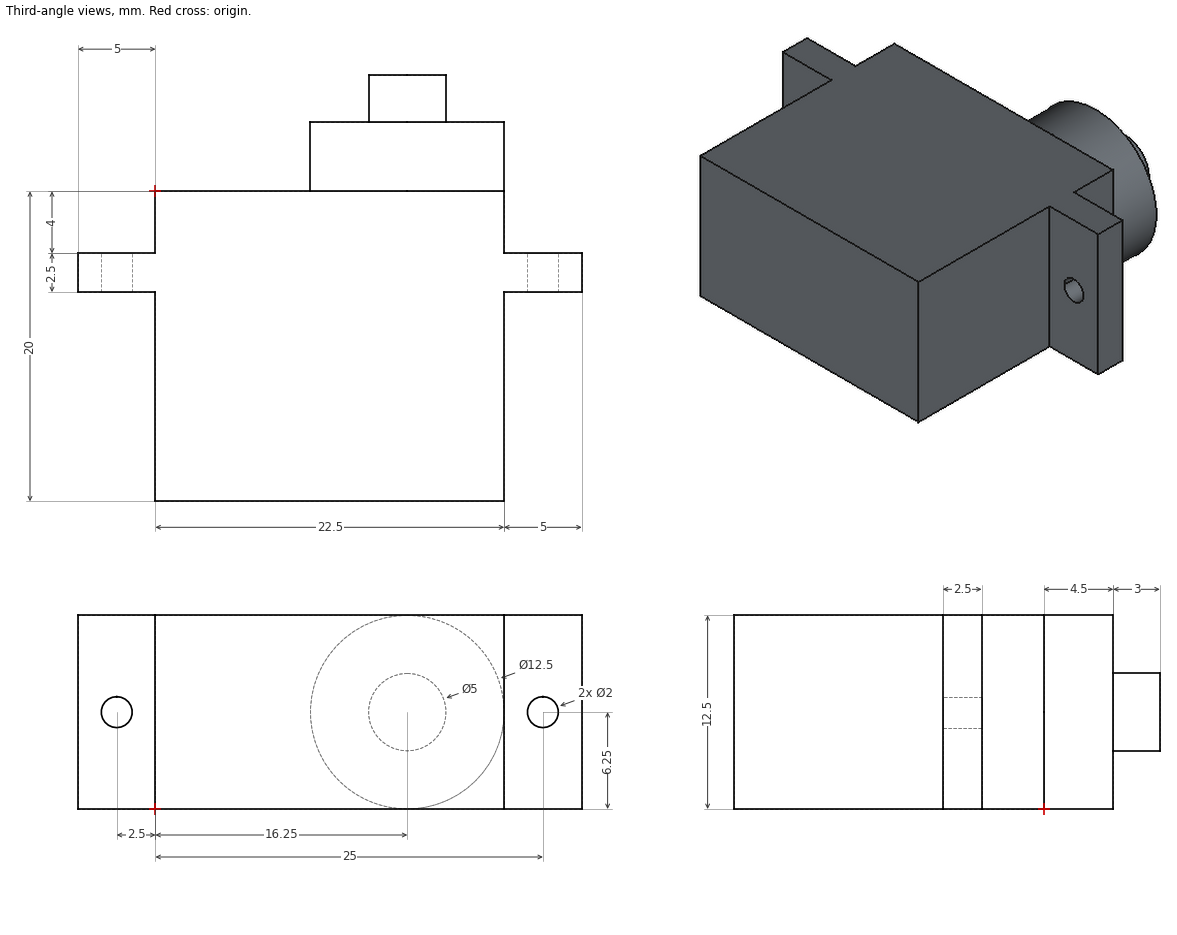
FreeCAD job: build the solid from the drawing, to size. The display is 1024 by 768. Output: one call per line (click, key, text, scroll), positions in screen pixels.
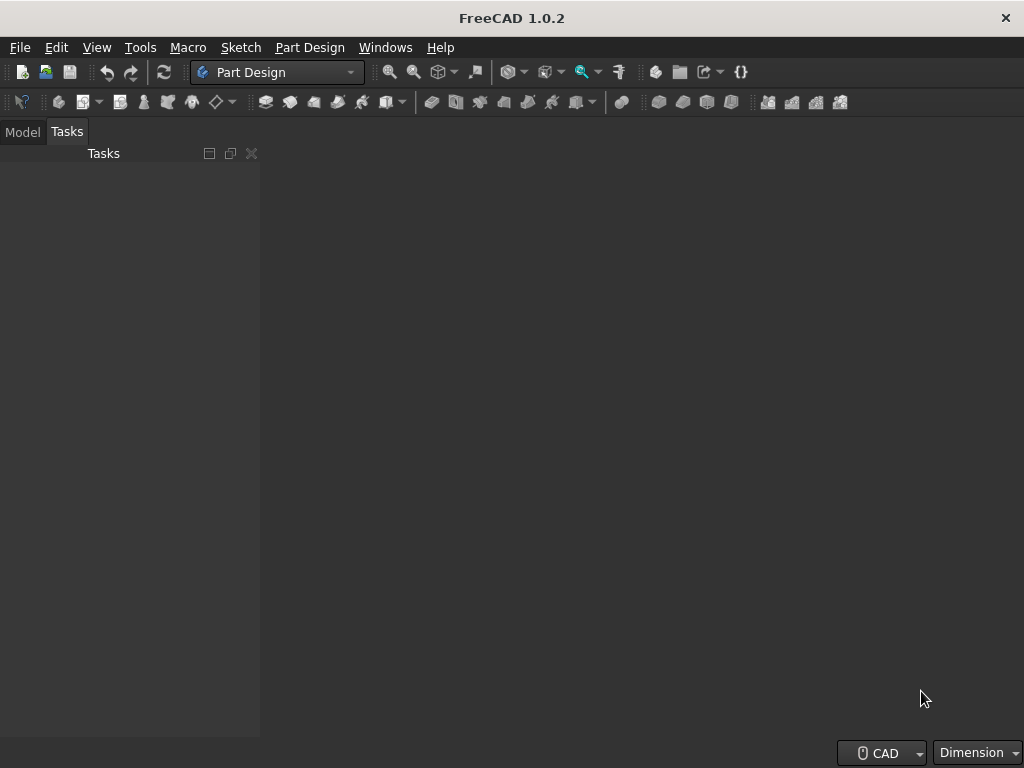
key(ctrl+n)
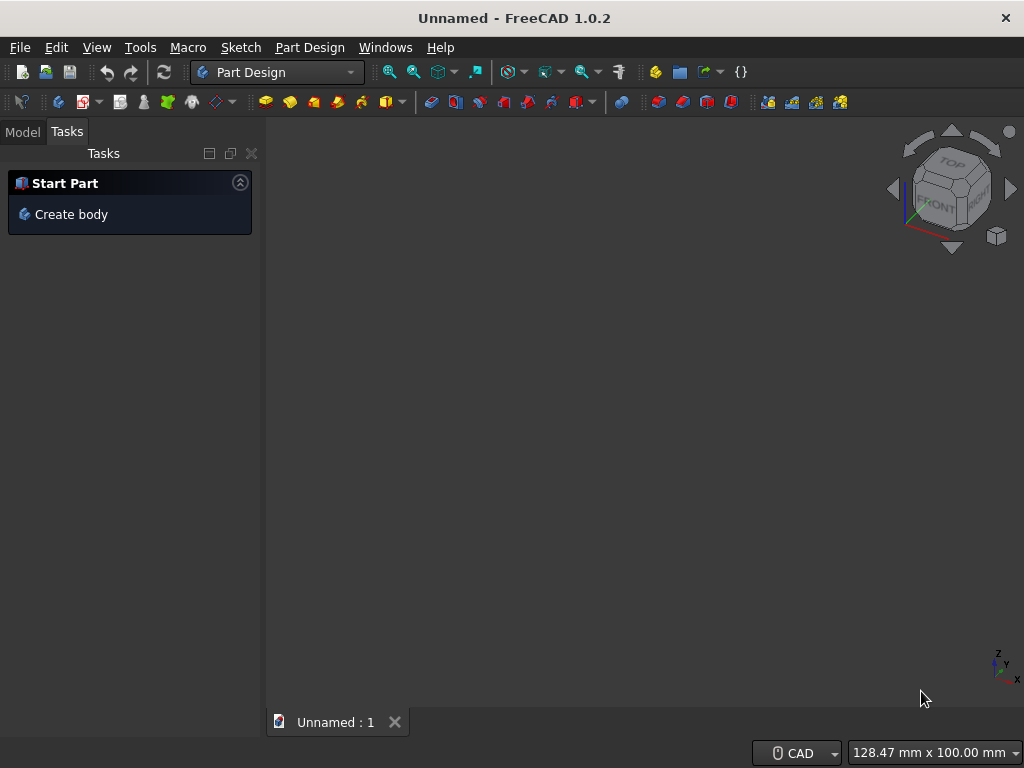
click(84, 102)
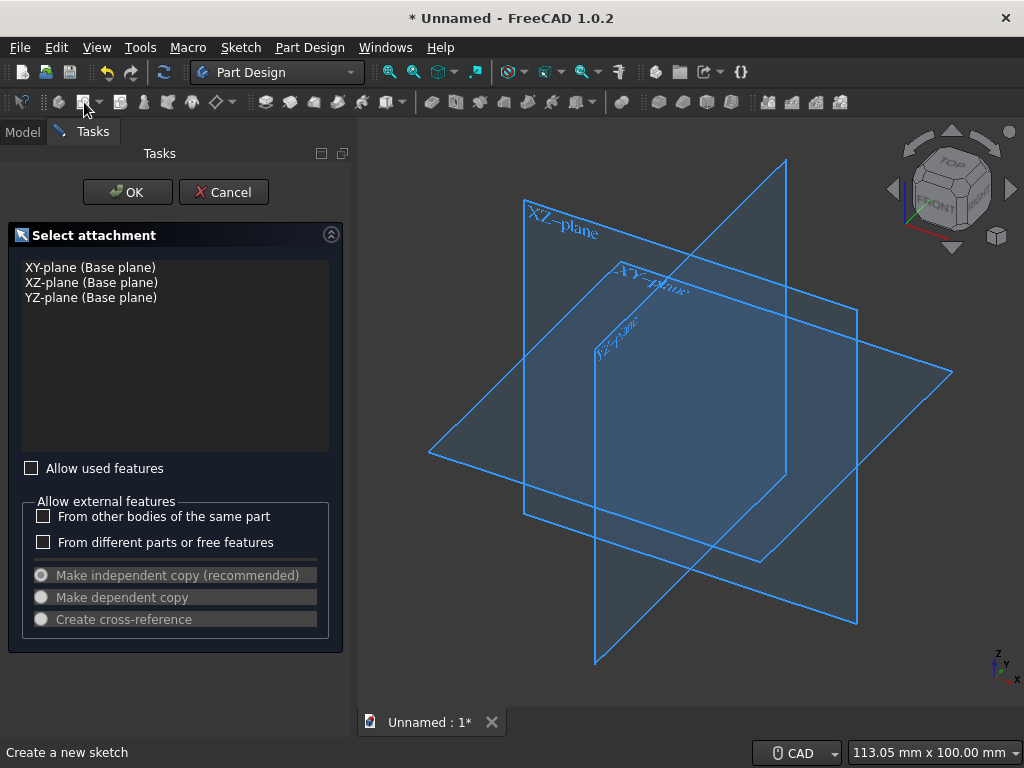
click(82, 268)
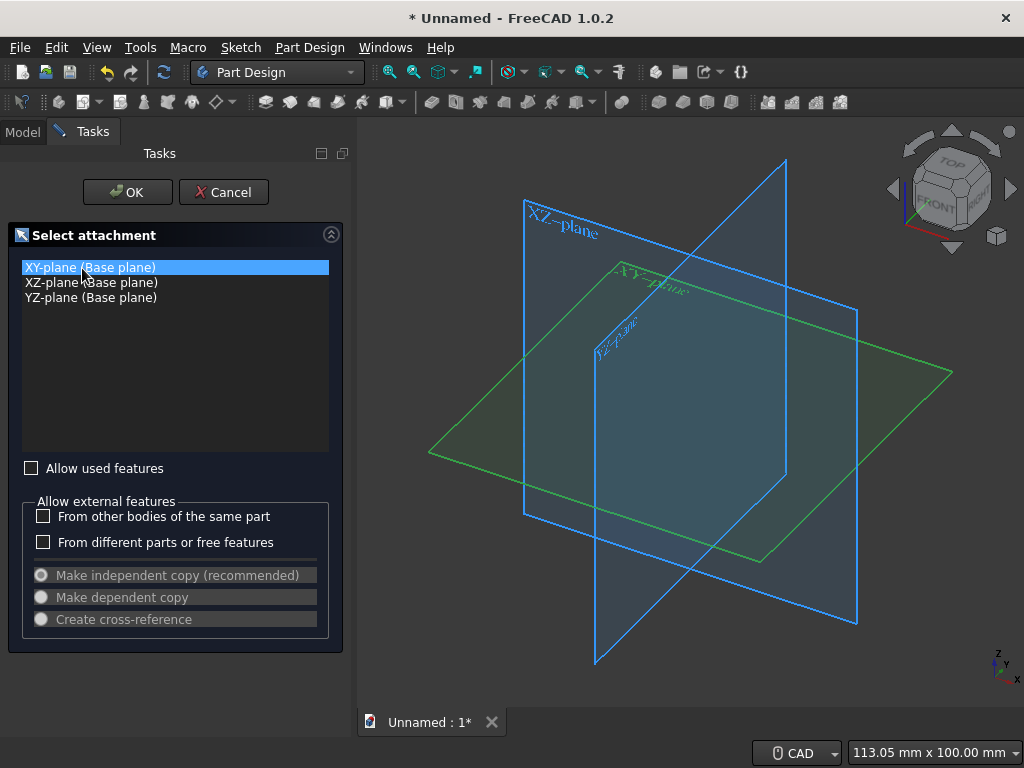
click(128, 192)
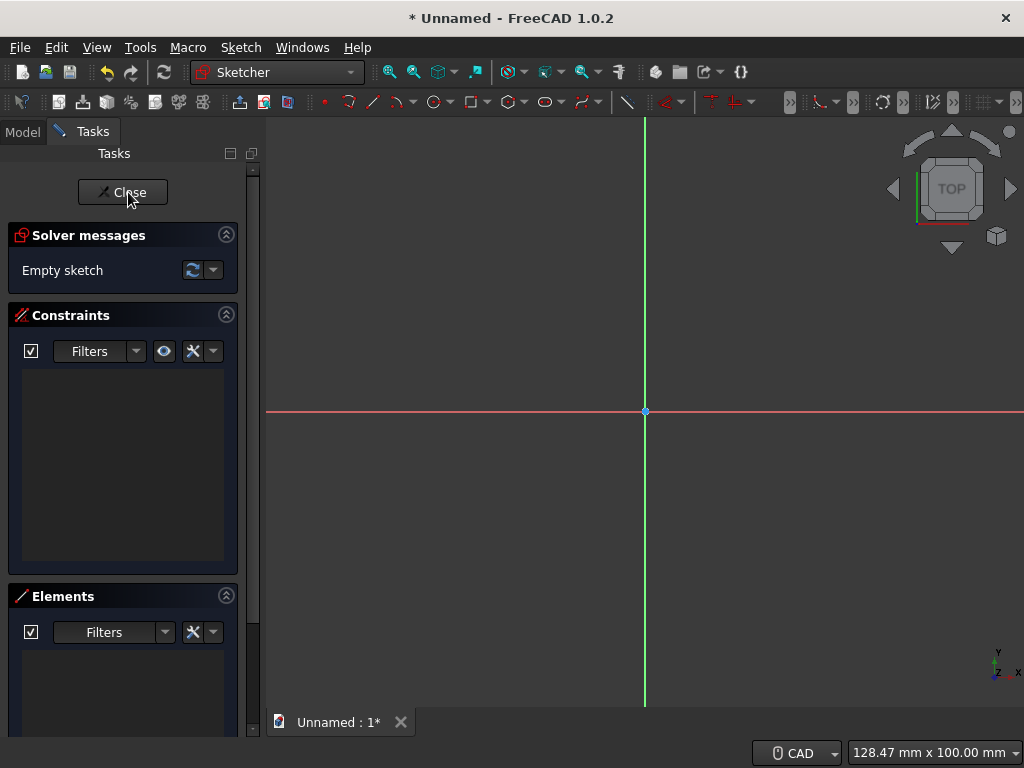
scroll(821, 519, up, 4)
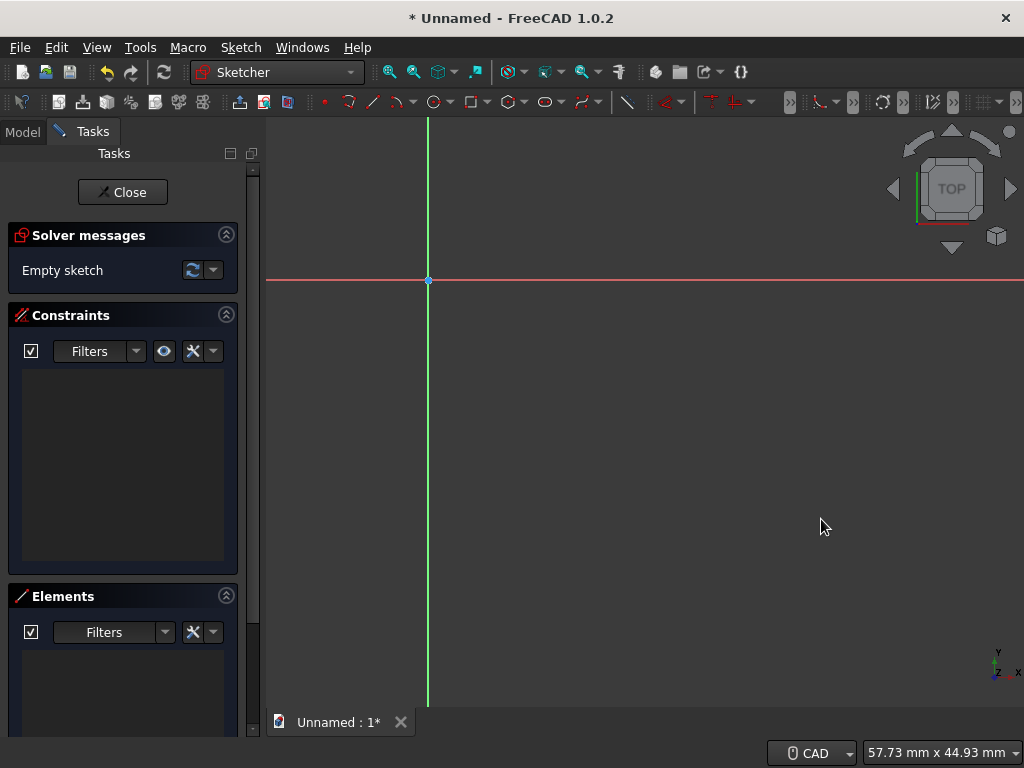
key(g)
key(m)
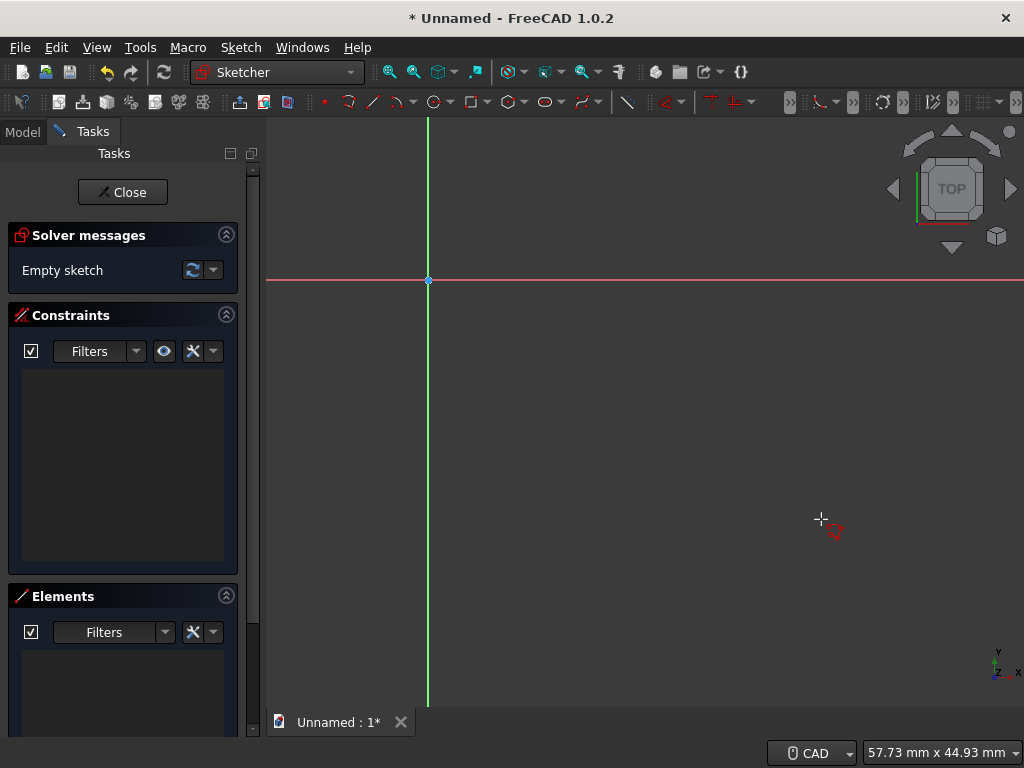
click(428, 280)
click(437, 333)
click(363, 333)
click(363, 365)
click(428, 365)
click(437, 543)
click(724, 543)
click(724, 365)
click(790, 365)
click(790, 333)
click(724, 333)
click(724, 289)
click(428, 280)
key(Escape)
key(Escape)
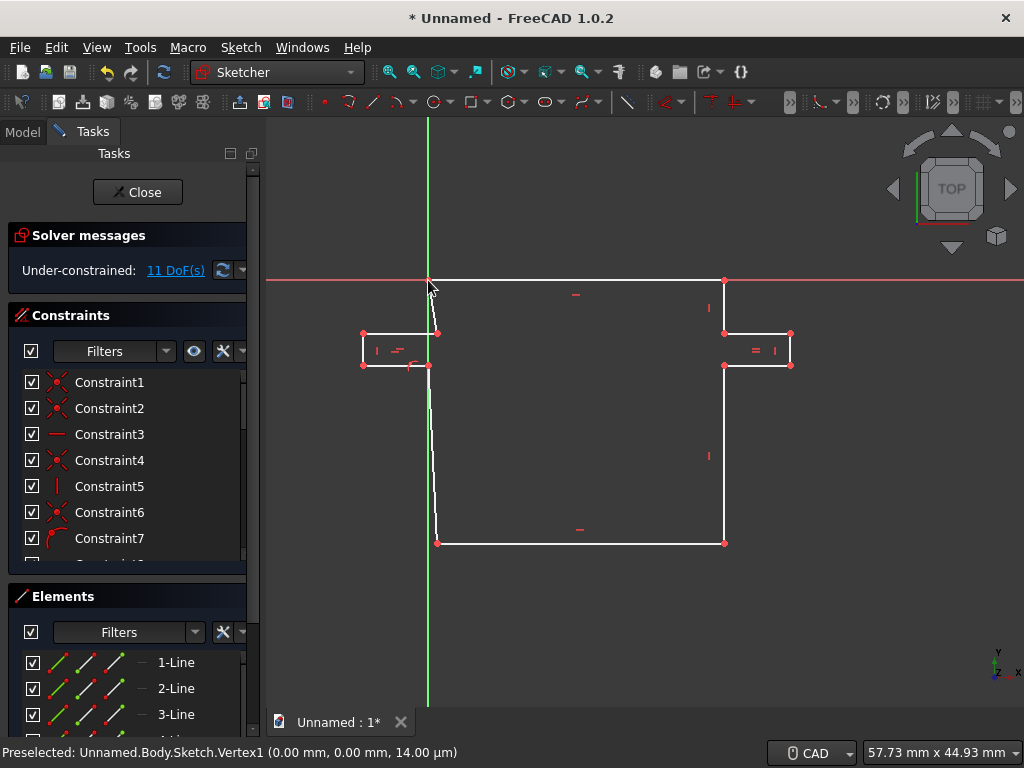
click(431, 296)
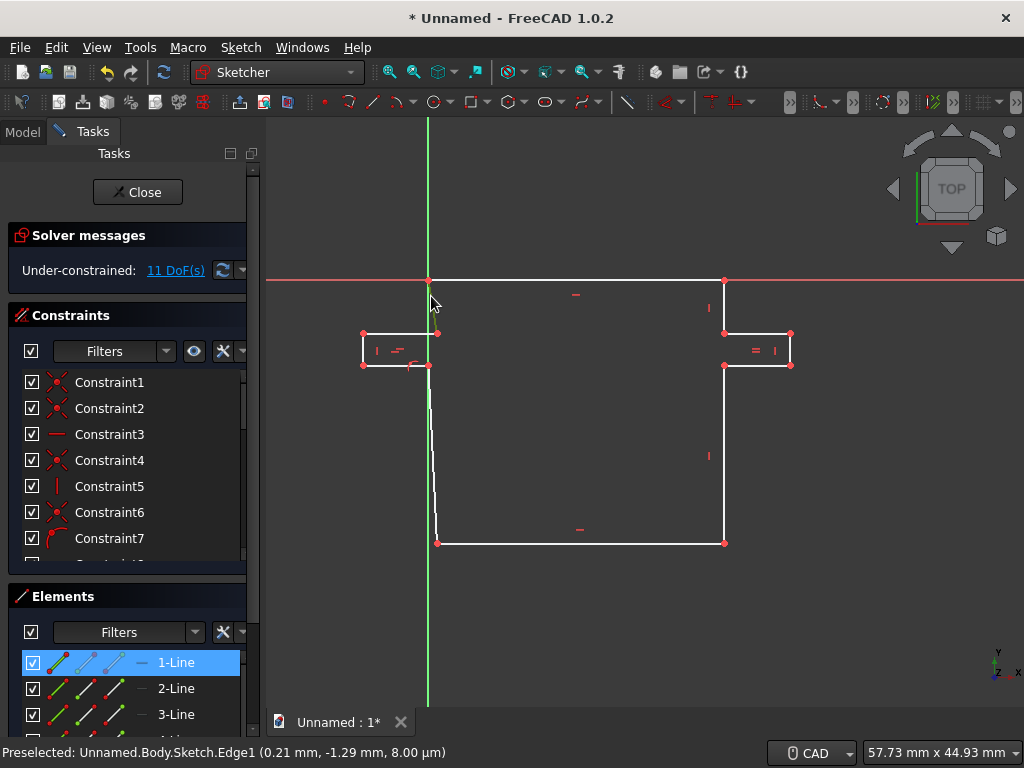
key(v)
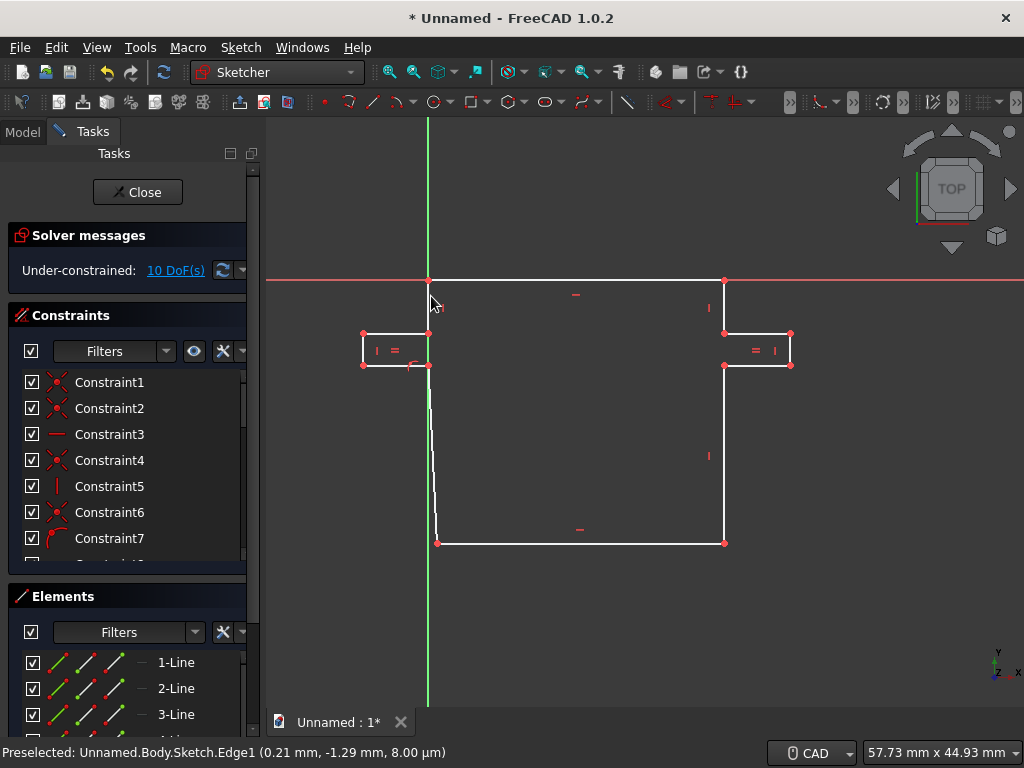
click(431, 419)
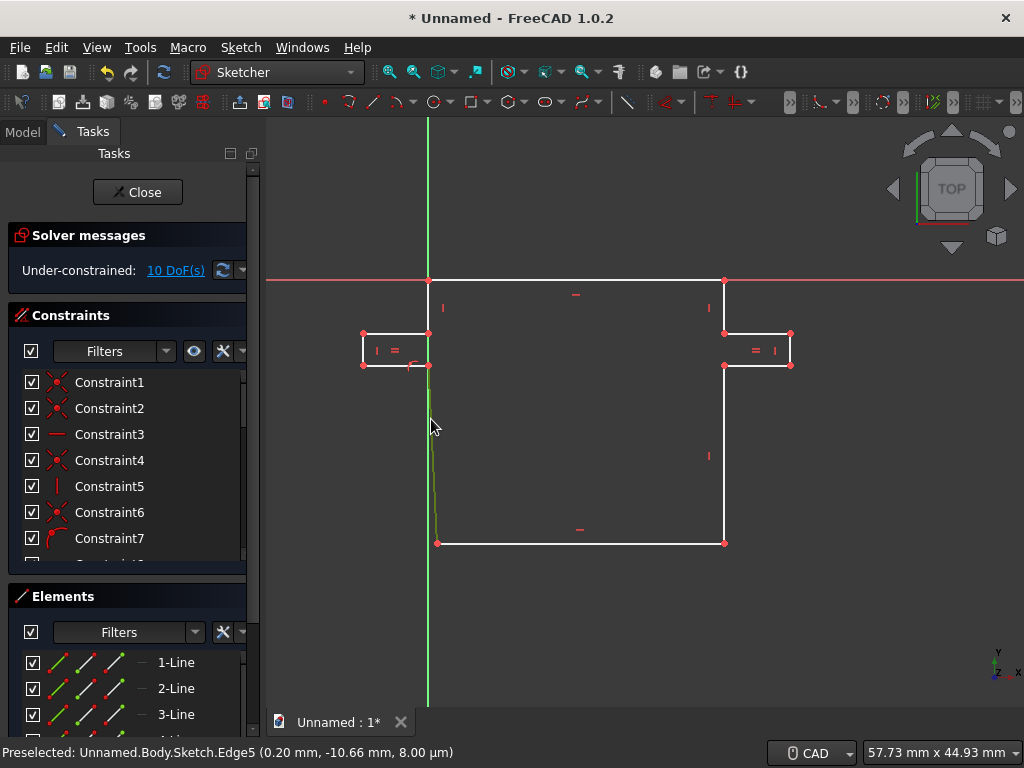
key(v)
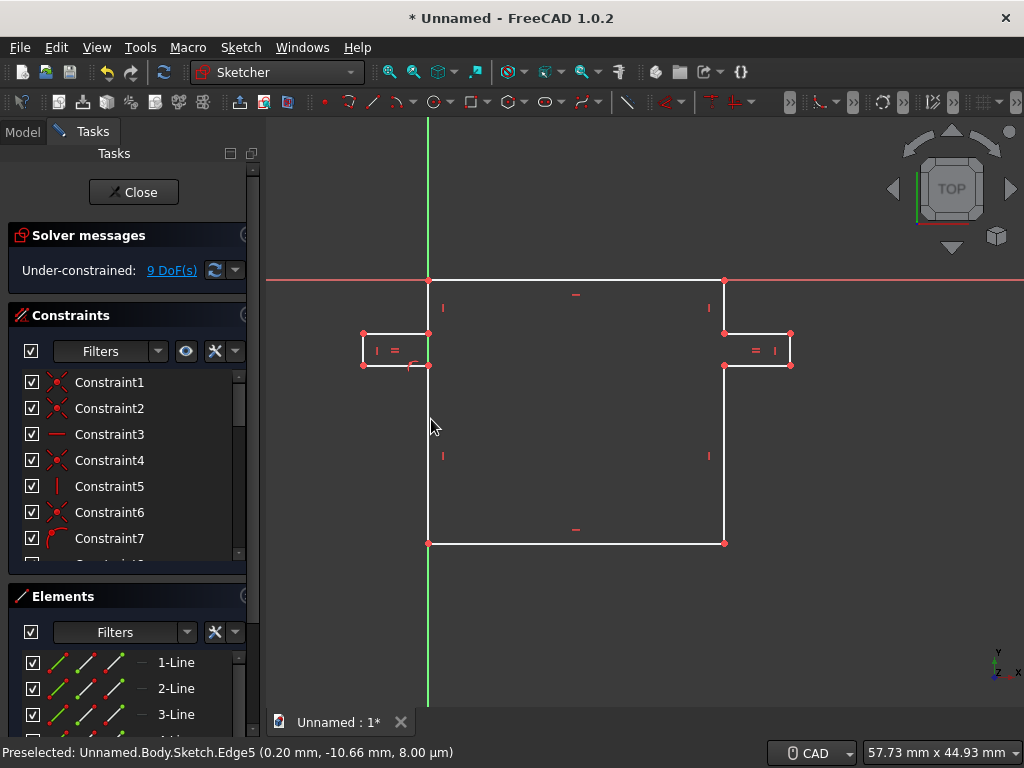
key(d)